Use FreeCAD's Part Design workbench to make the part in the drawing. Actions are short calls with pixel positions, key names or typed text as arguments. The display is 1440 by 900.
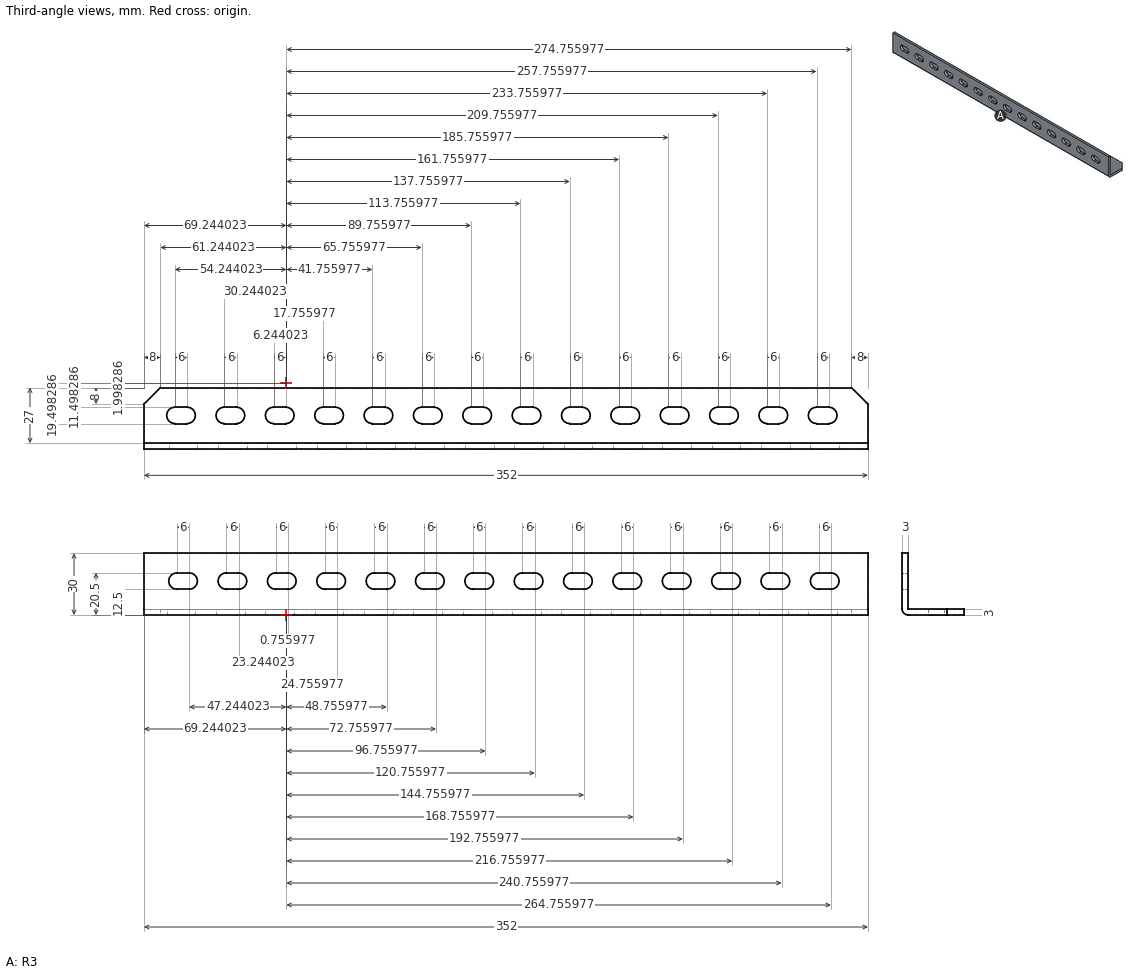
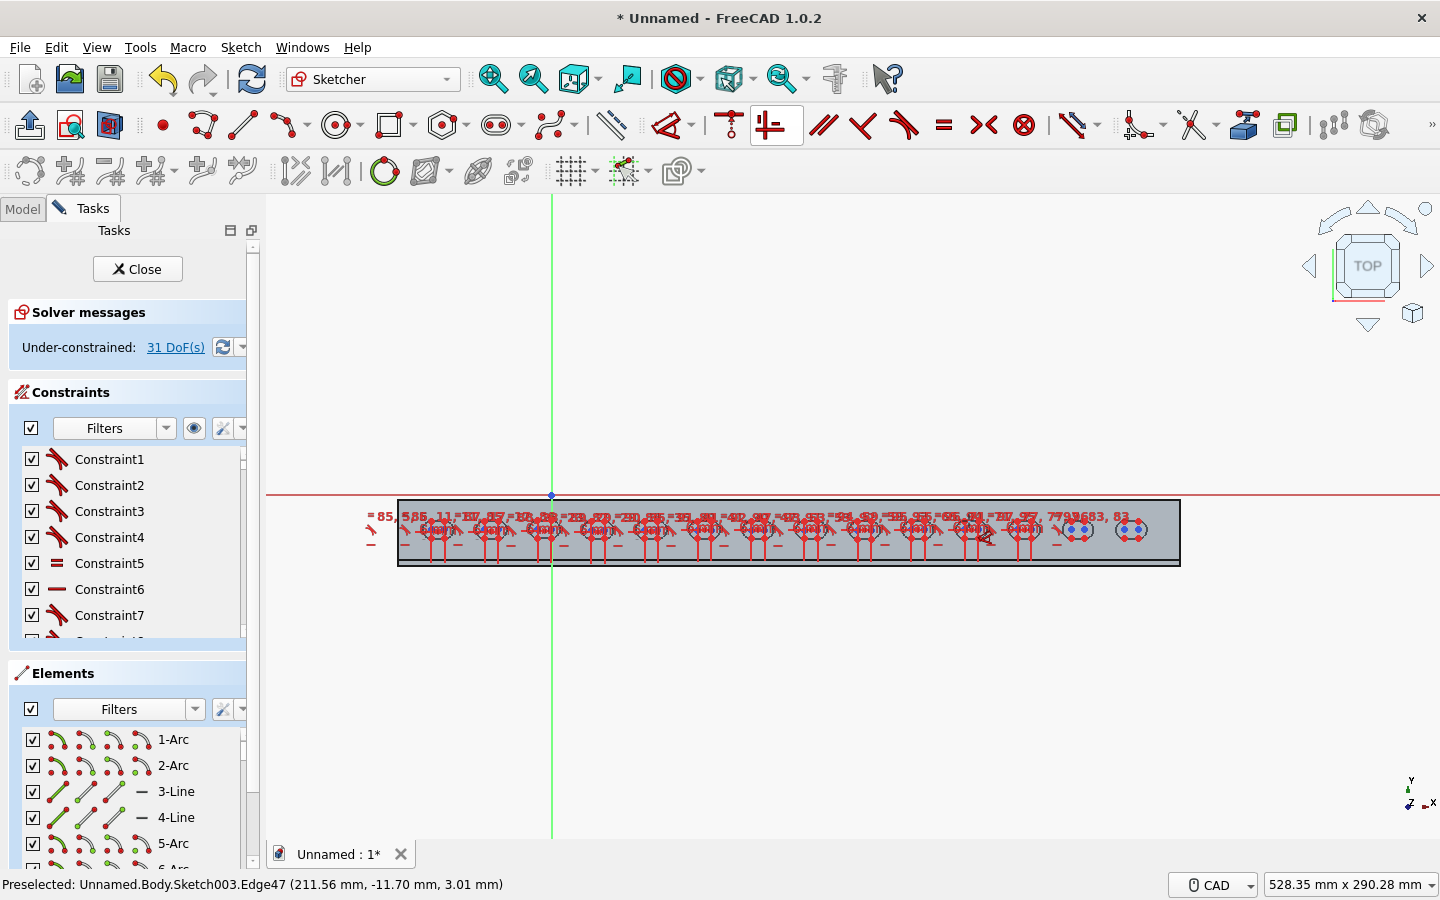
scroll(1075, 521, up, 7)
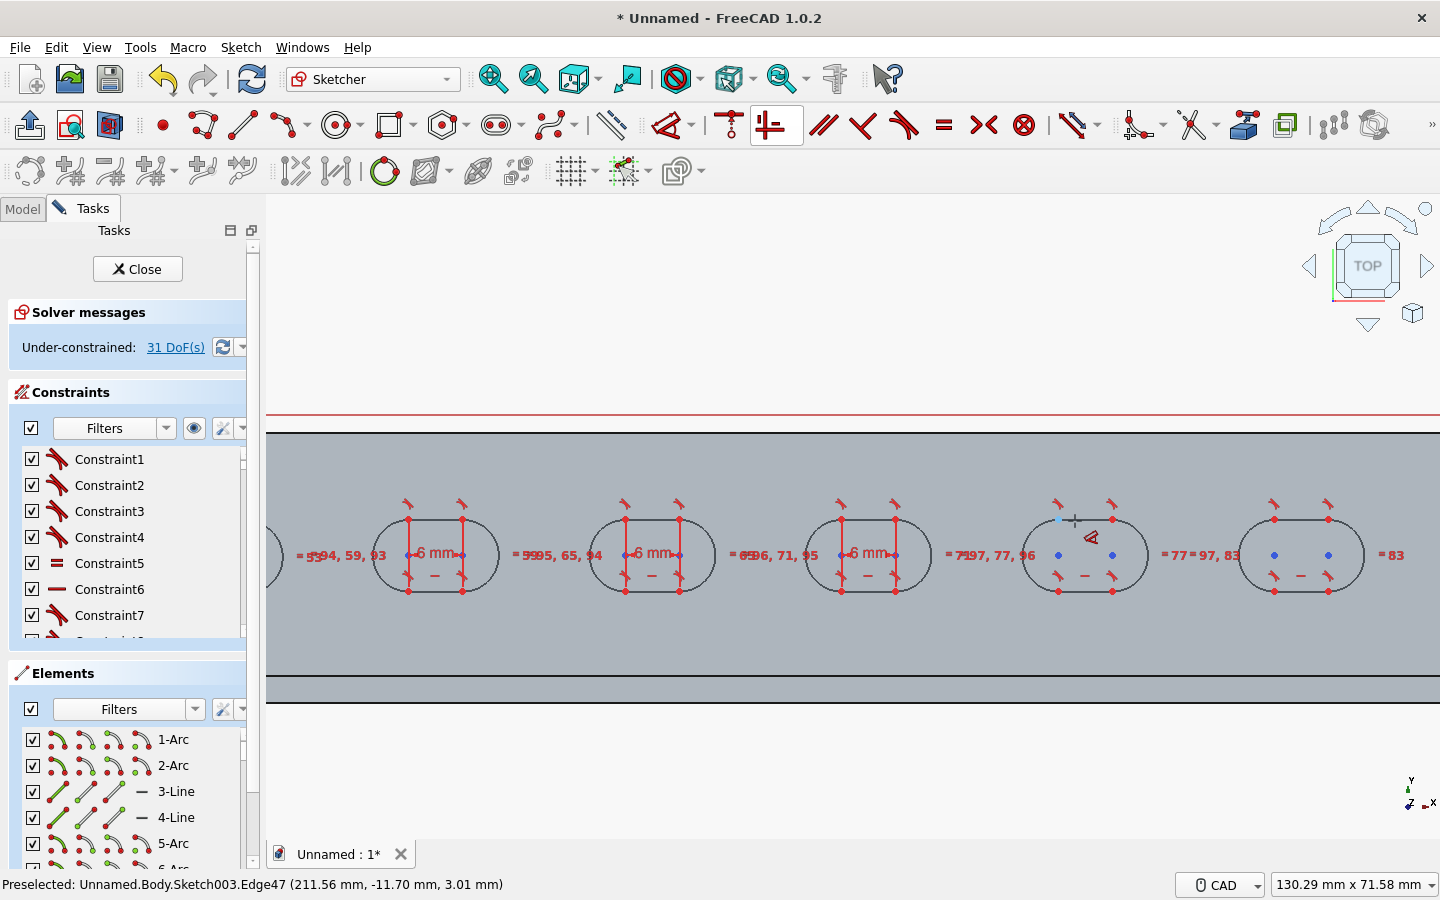
click(1075, 520)
click(1085, 554)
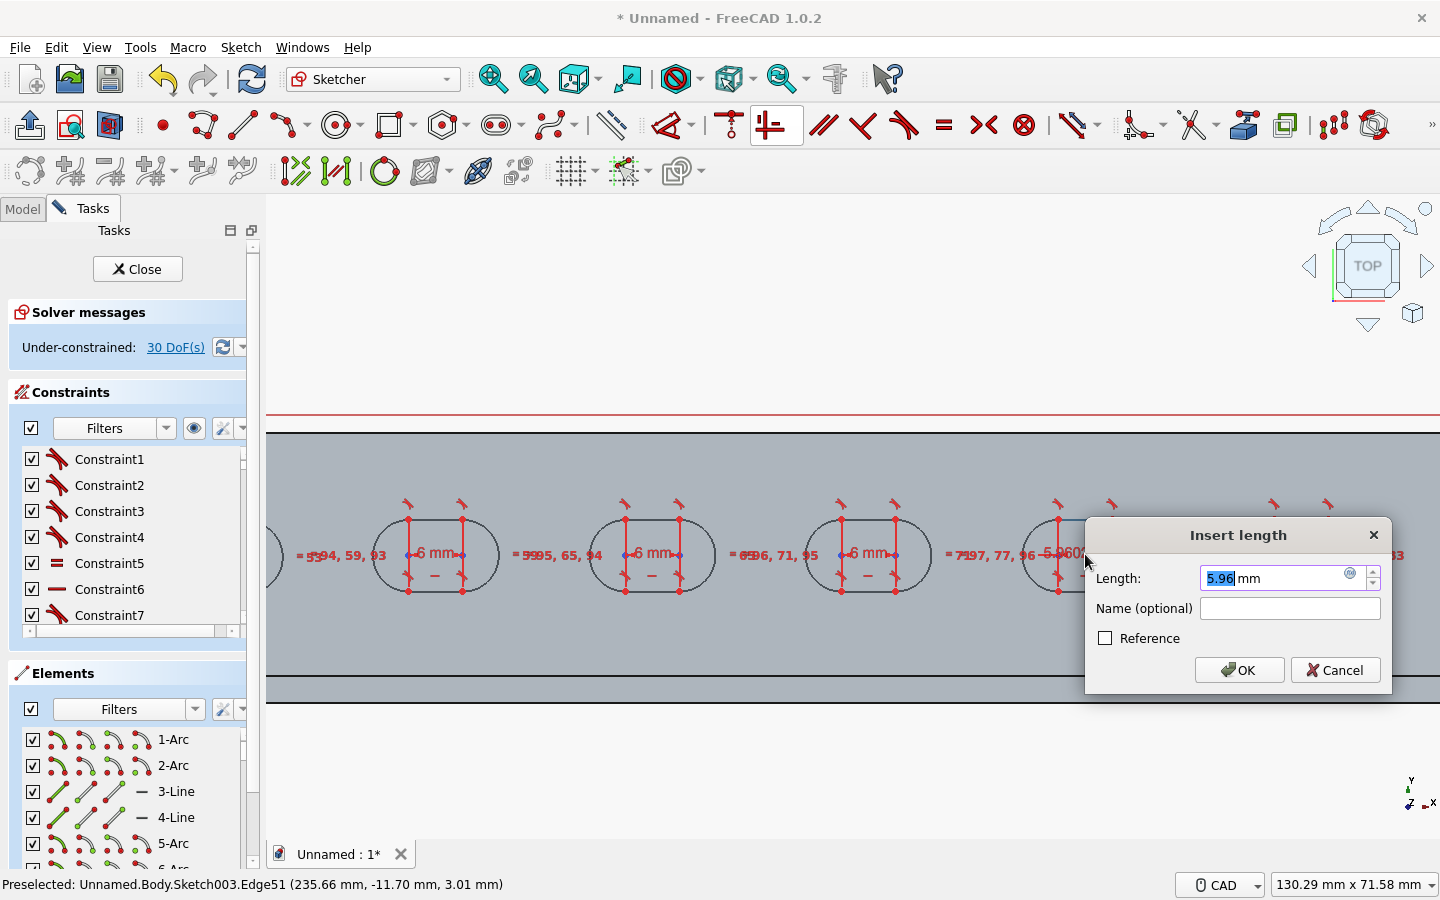
text(6)
key(Return)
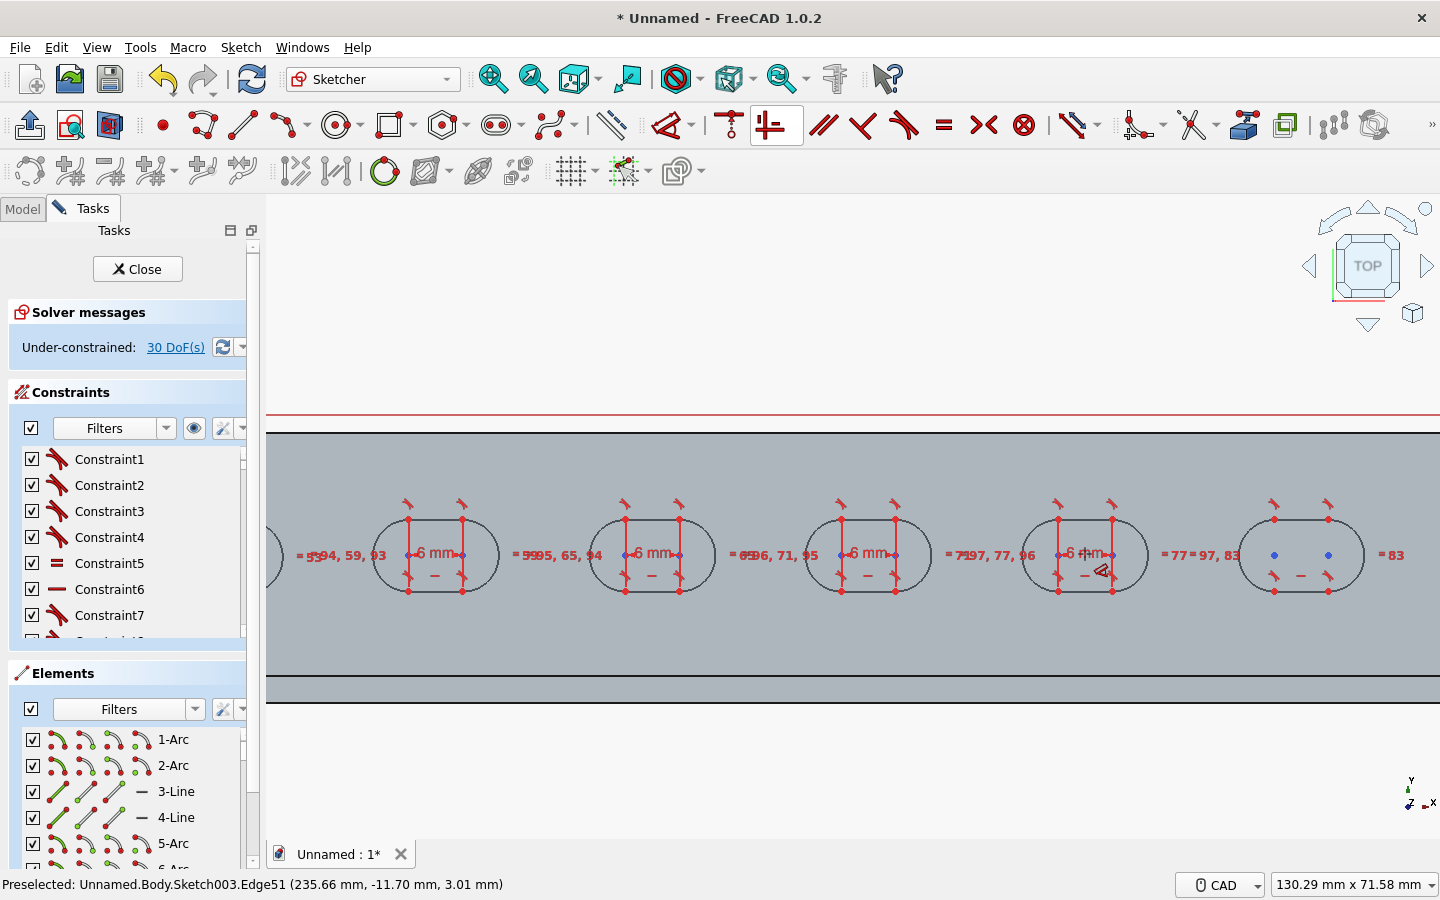
scroll(1075, 521, down, 7)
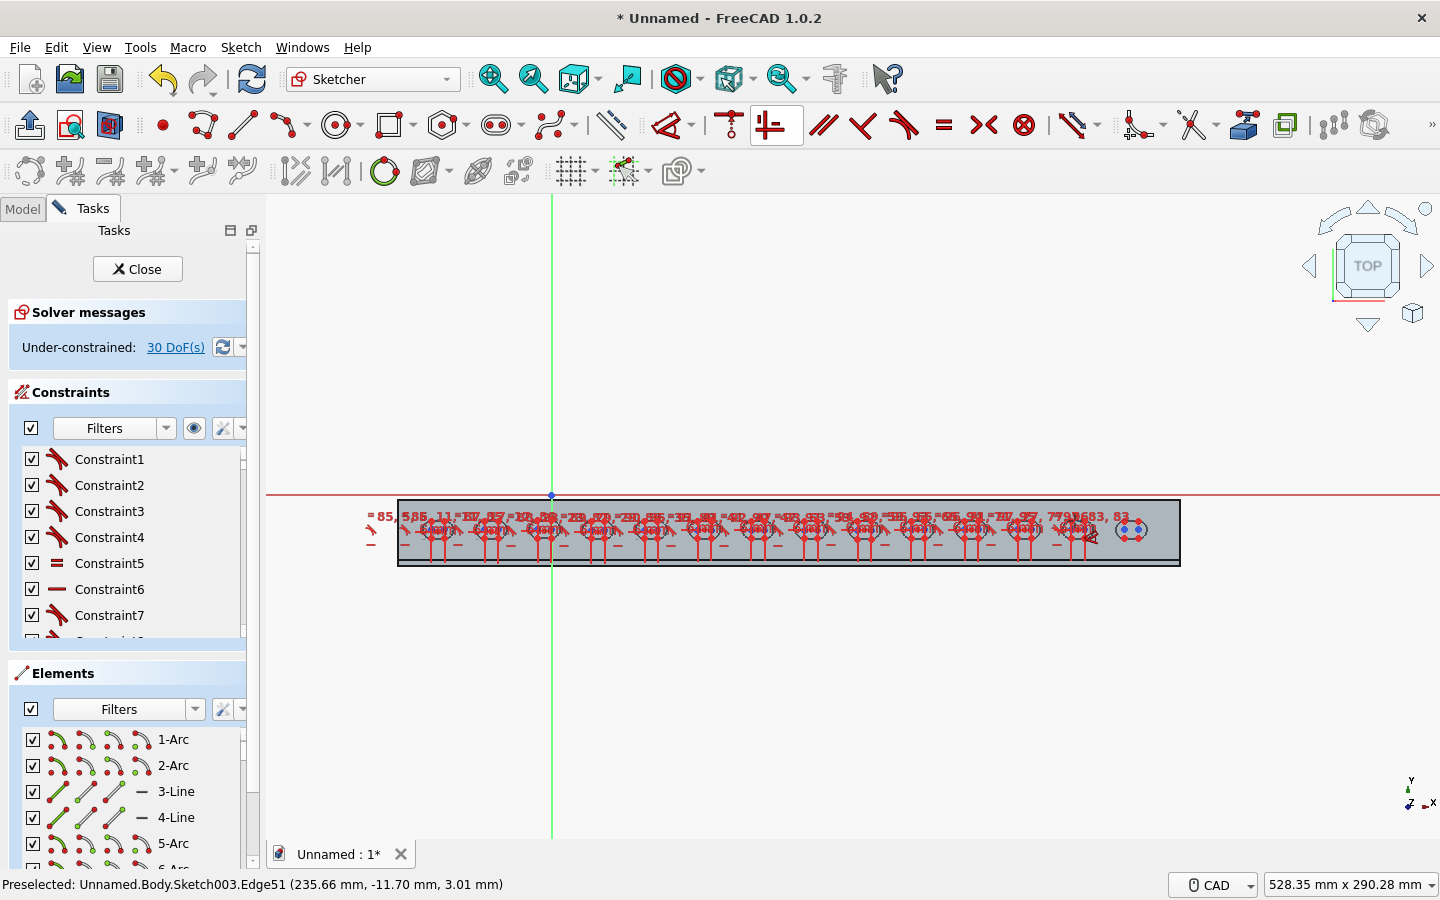
scroll(1129, 521, up, 7)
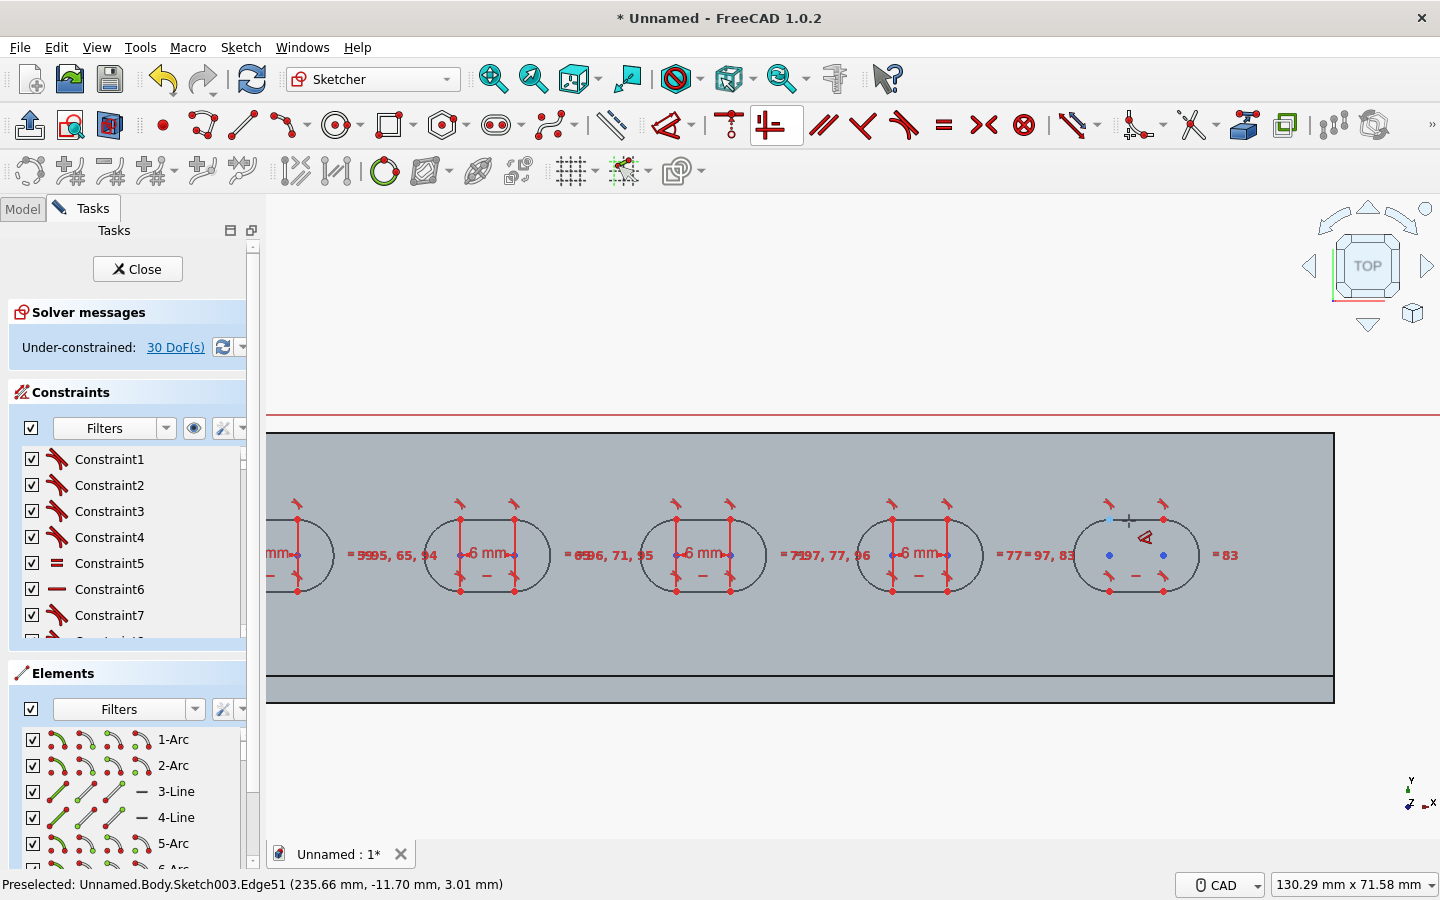
click(1126, 520)
click(1136, 554)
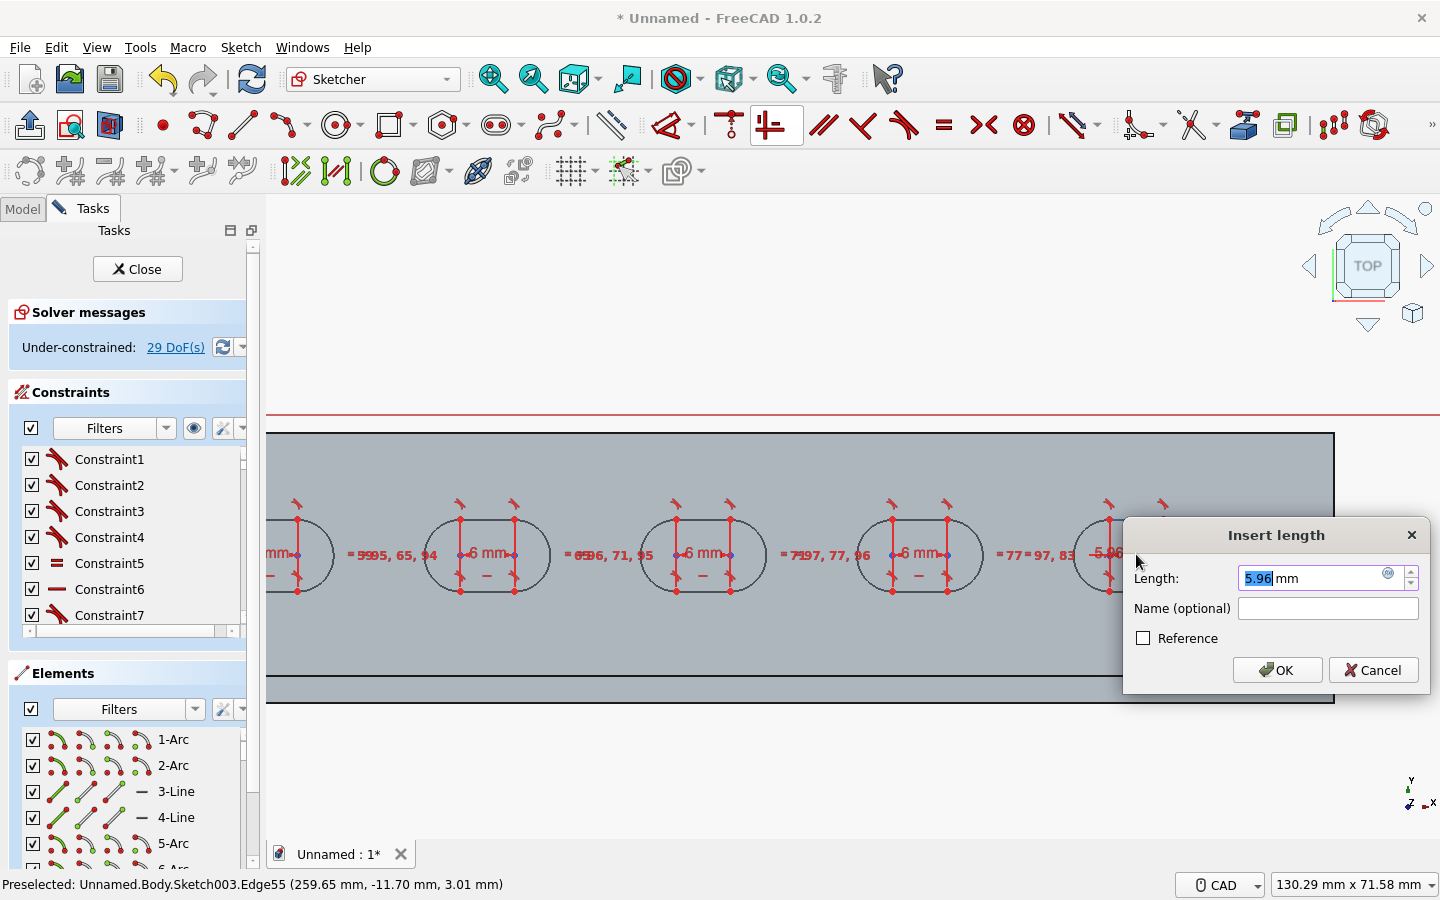
text(6)
key(Return)